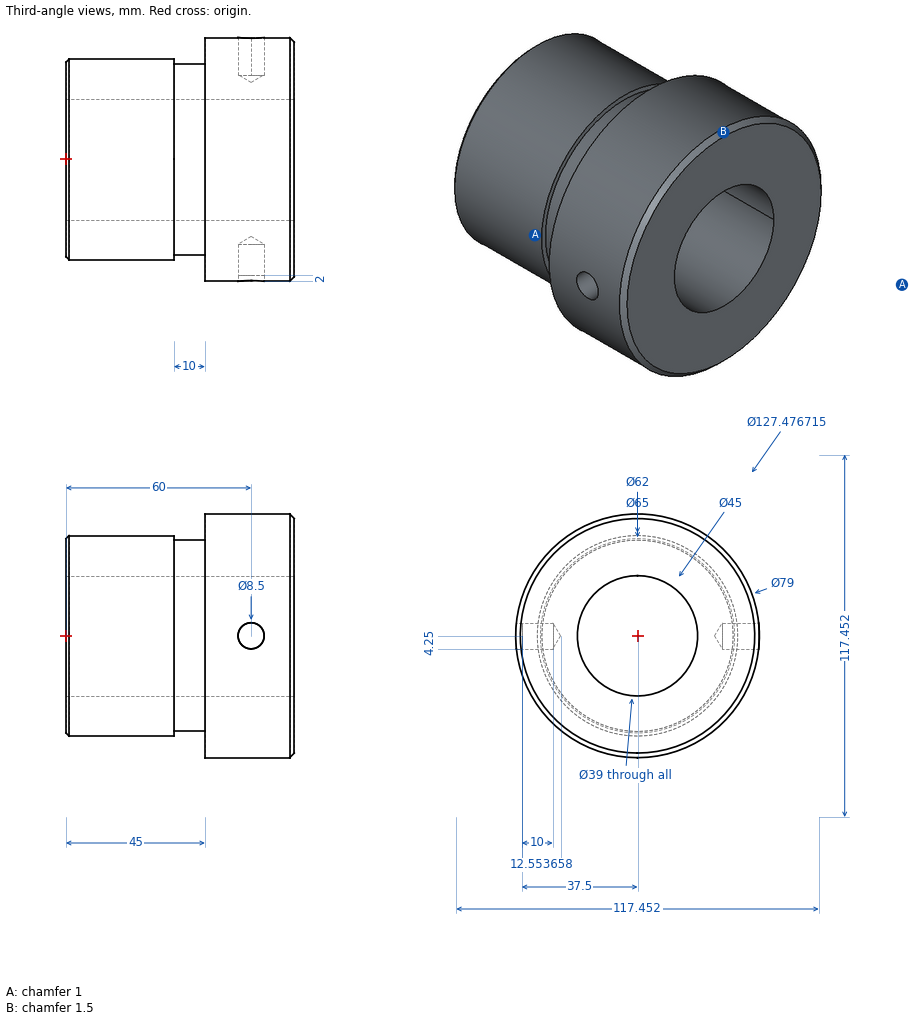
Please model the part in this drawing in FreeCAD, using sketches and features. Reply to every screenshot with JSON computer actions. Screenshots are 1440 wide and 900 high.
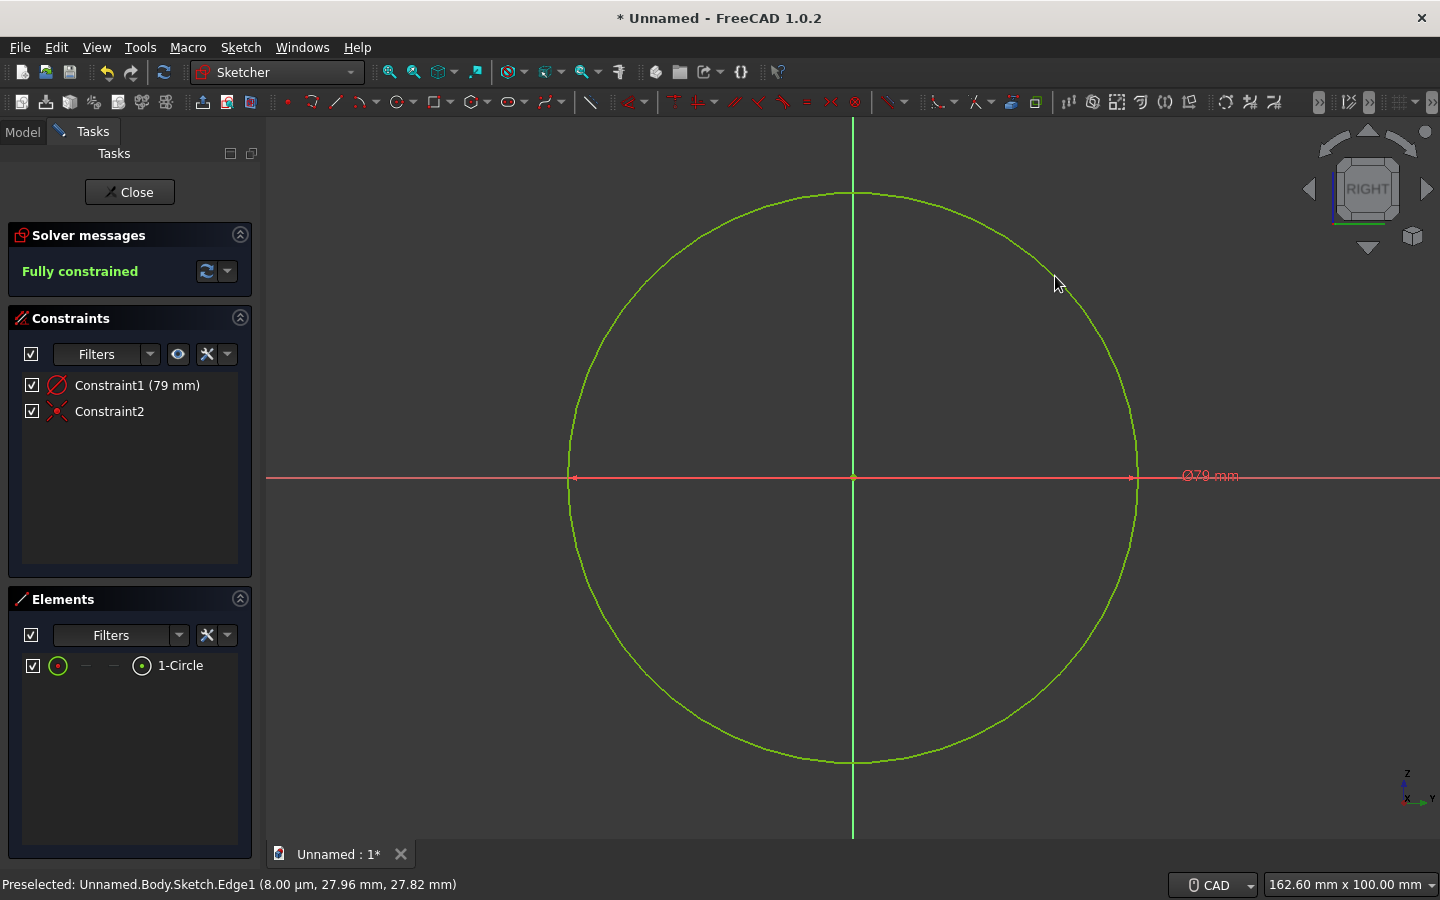
{"action": "left_click", "coordinate": [130, 192]}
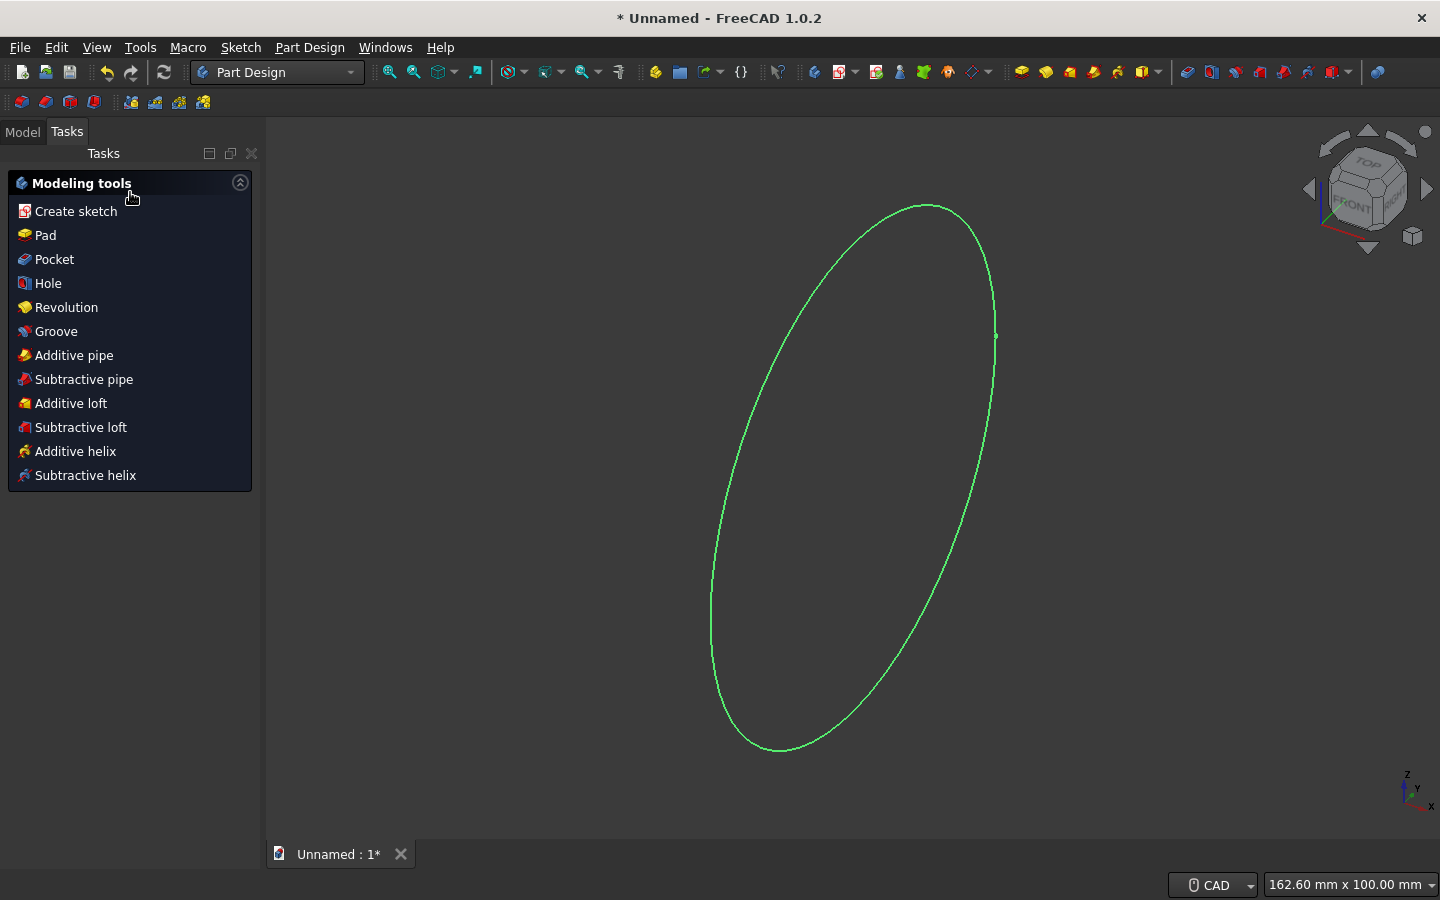
{"action": "left_click", "coordinate": [1022, 72]}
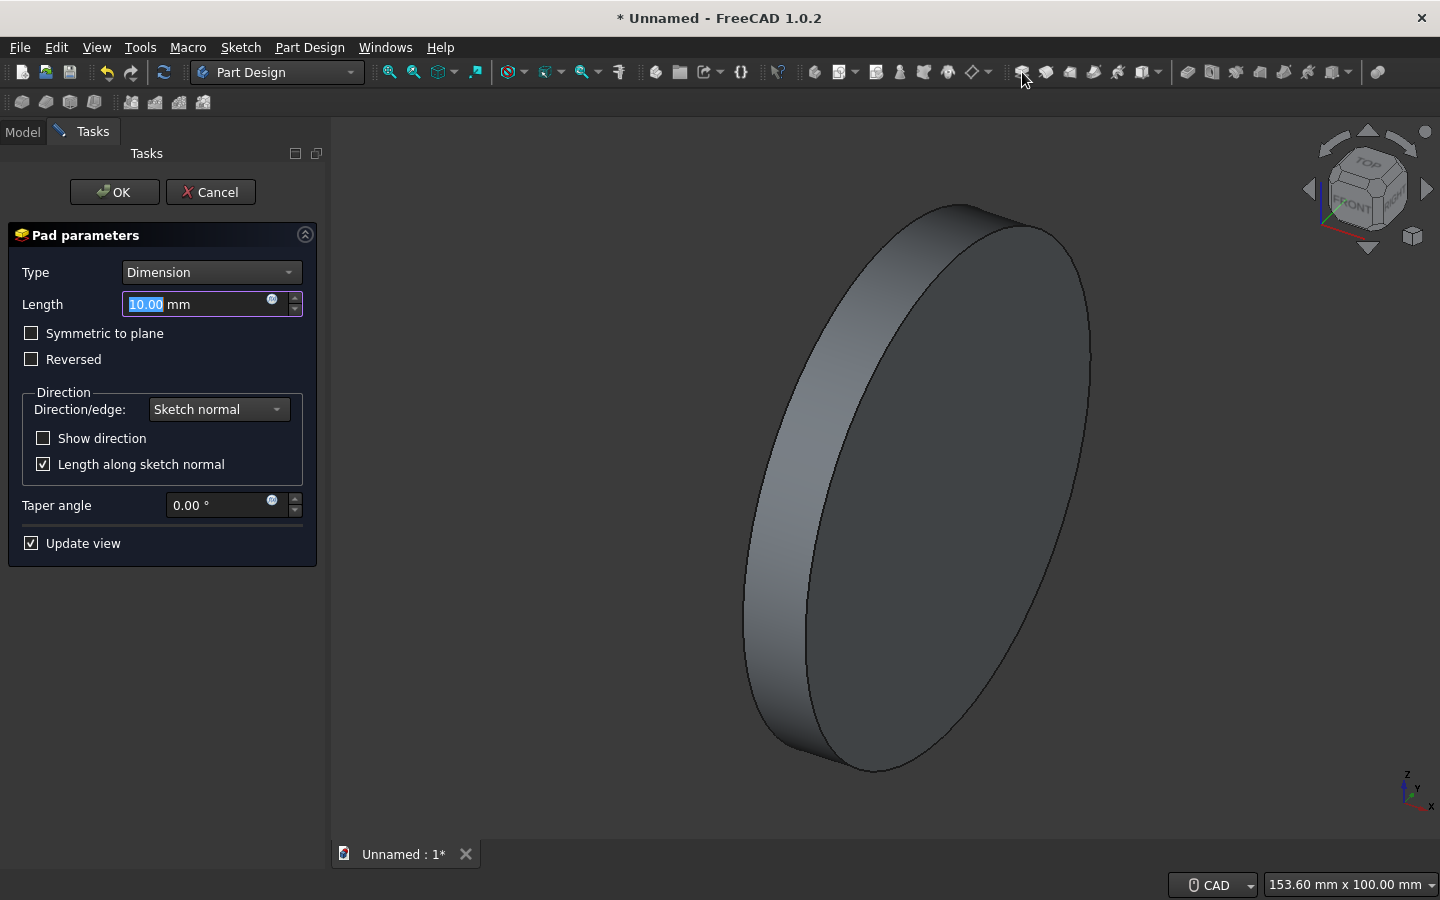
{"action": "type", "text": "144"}
{"action": "key", "text": "Tab"}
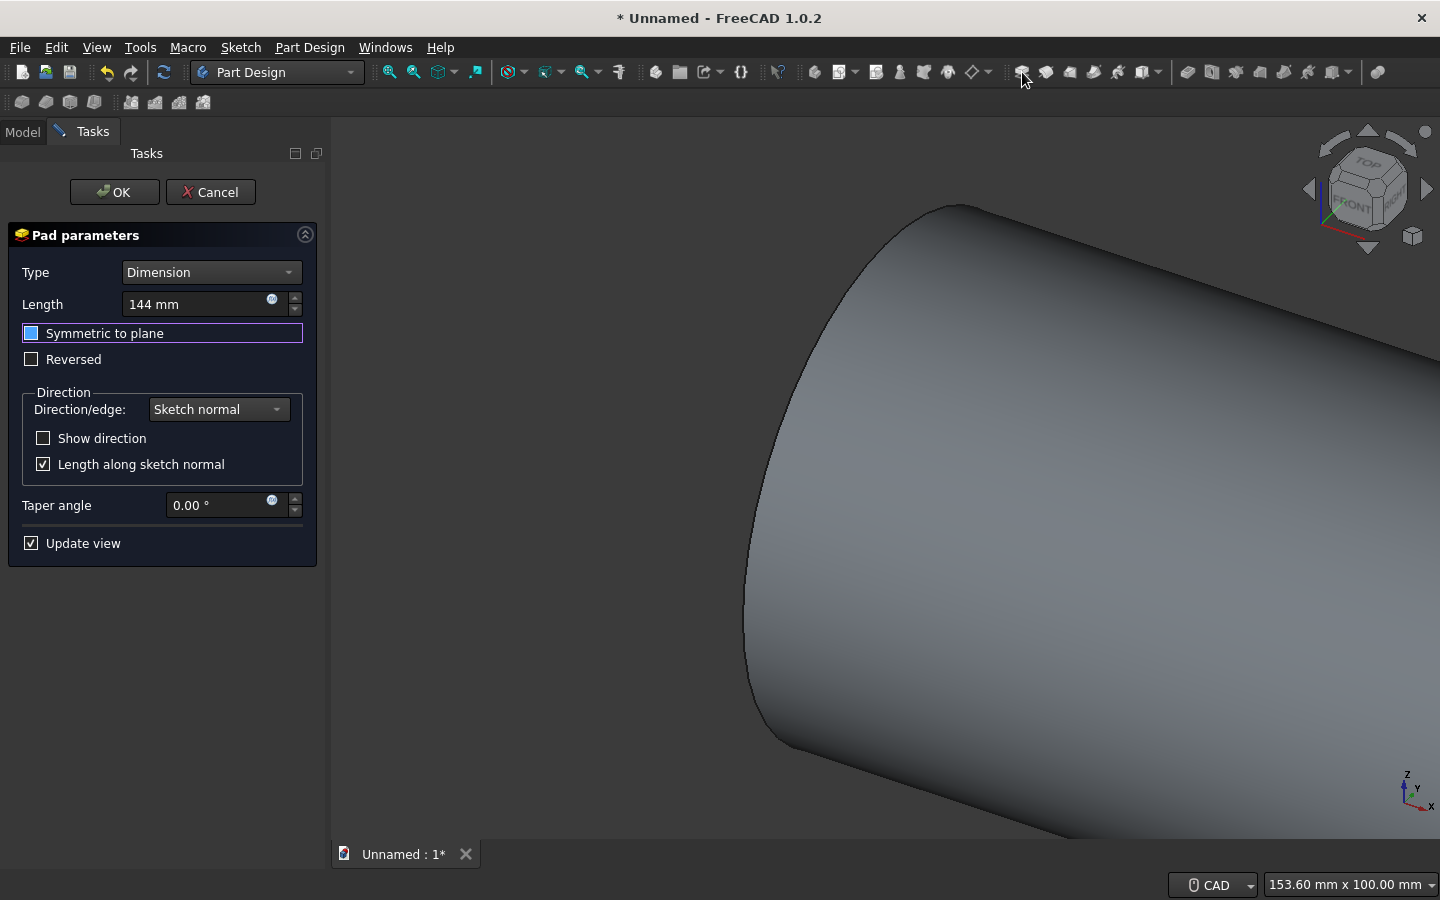
{"action": "left_click", "coordinate": [115, 192]}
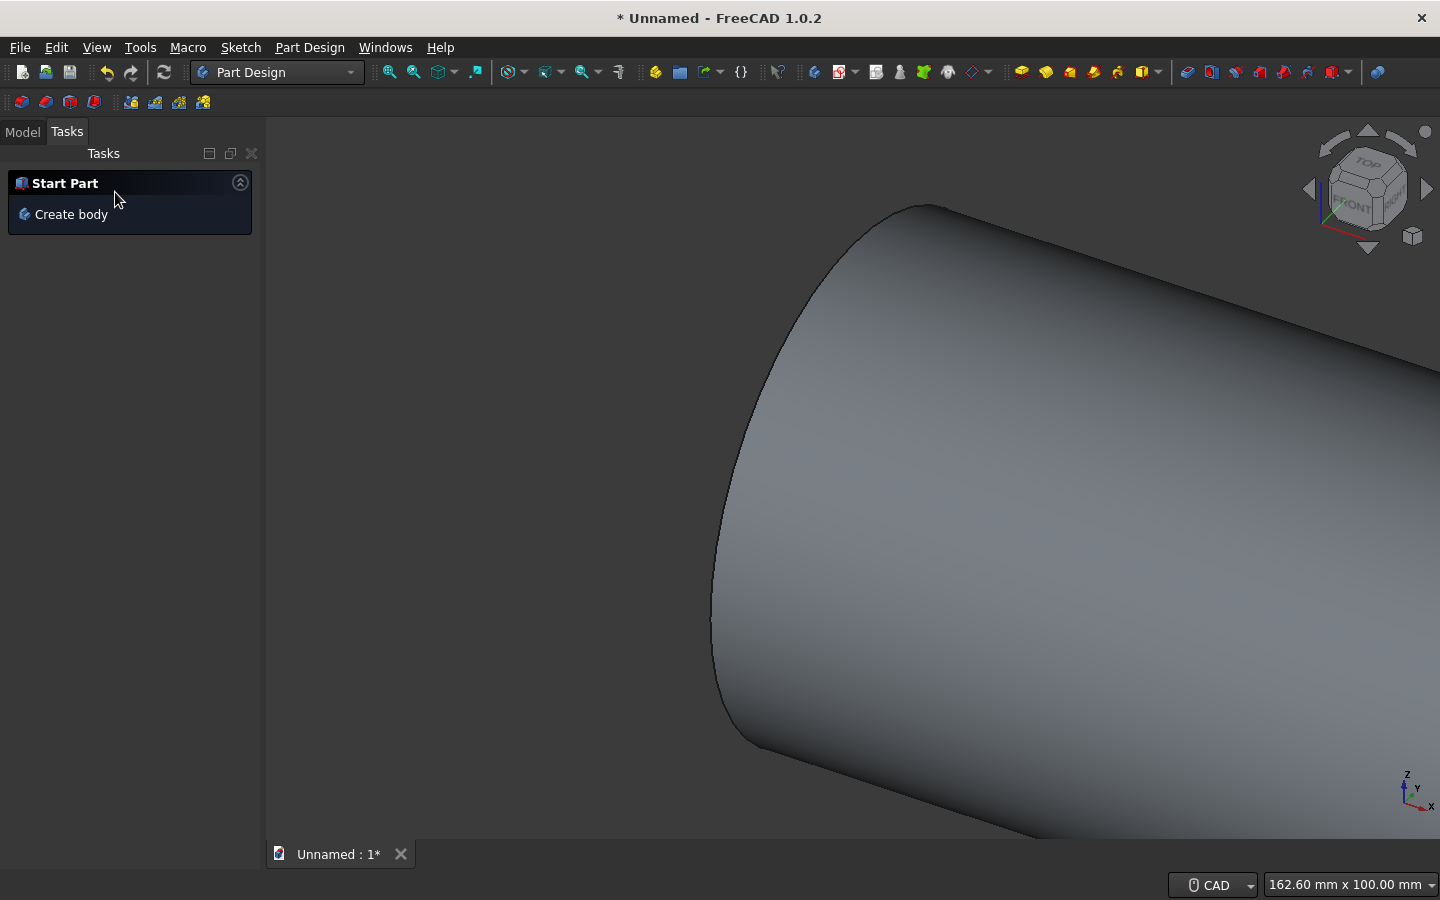
{"action": "key", "text": "v f"}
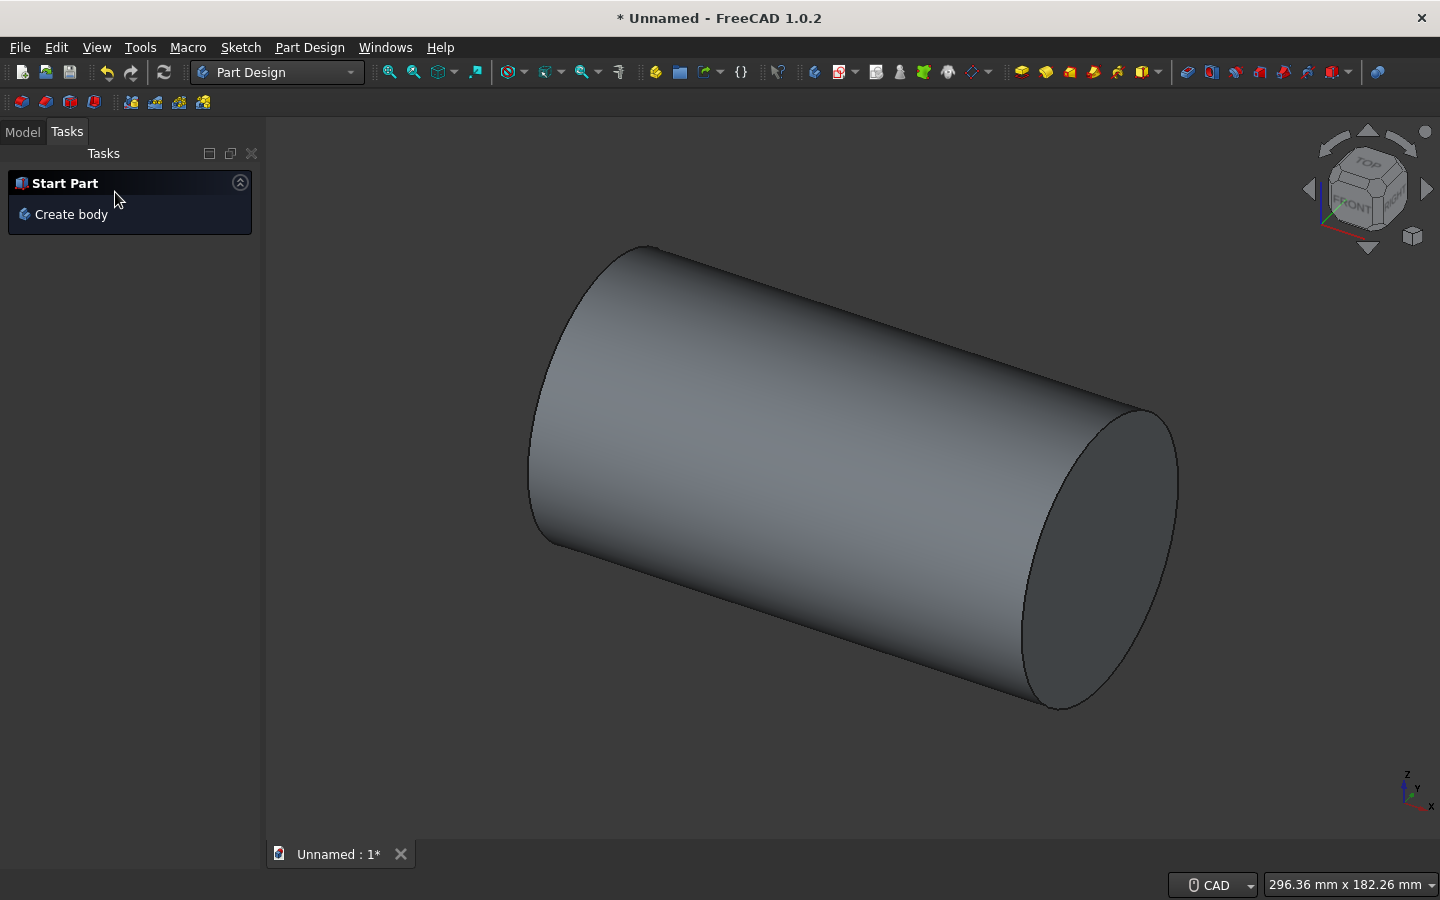
{"action": "left_click", "coordinate": [1100, 559]}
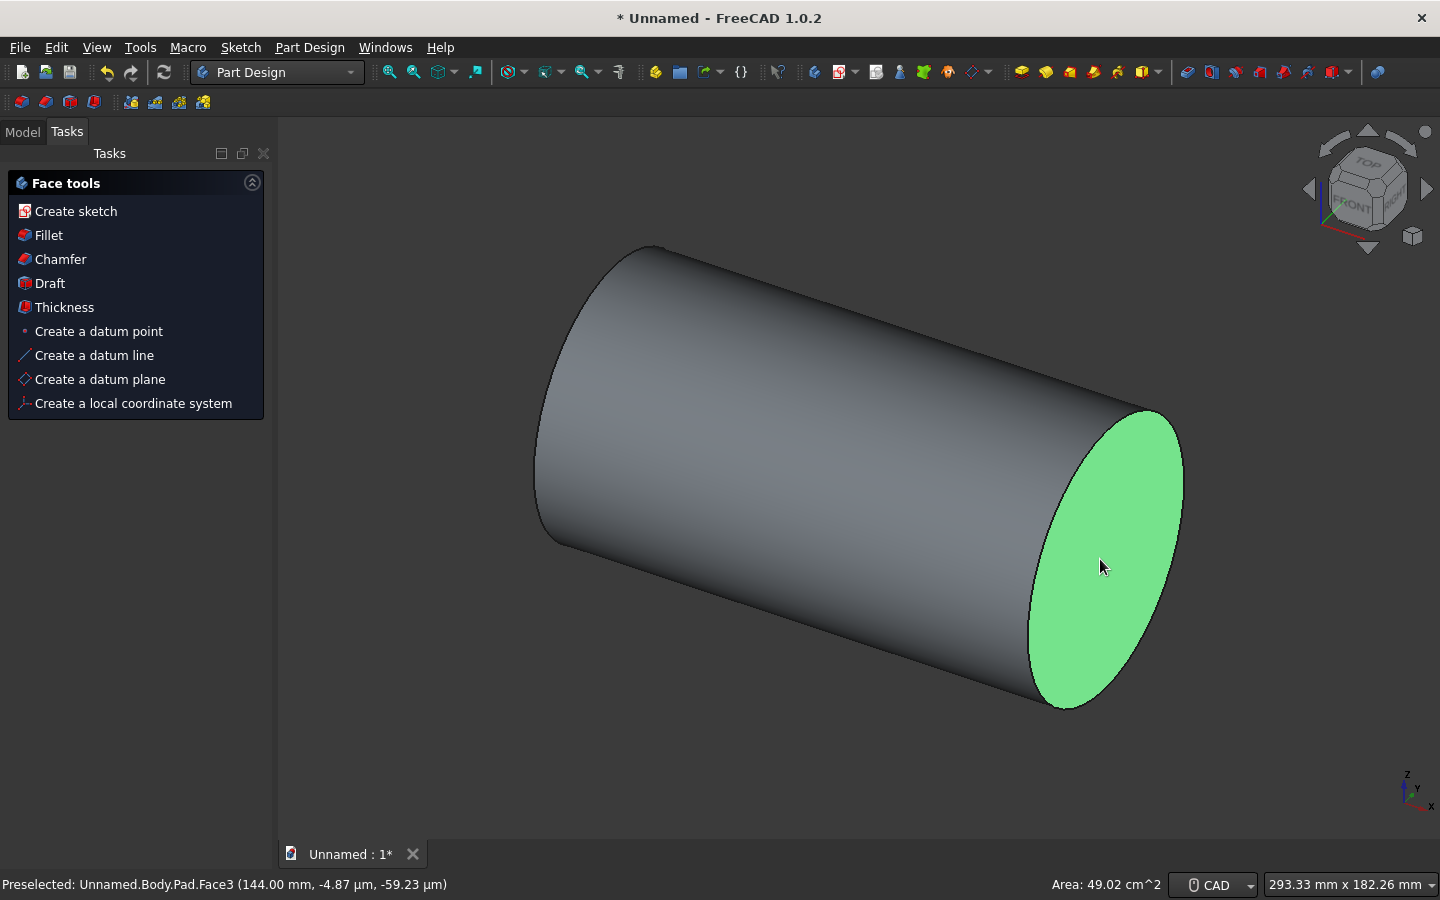
{"action": "left_click", "coordinate": [840, 72]}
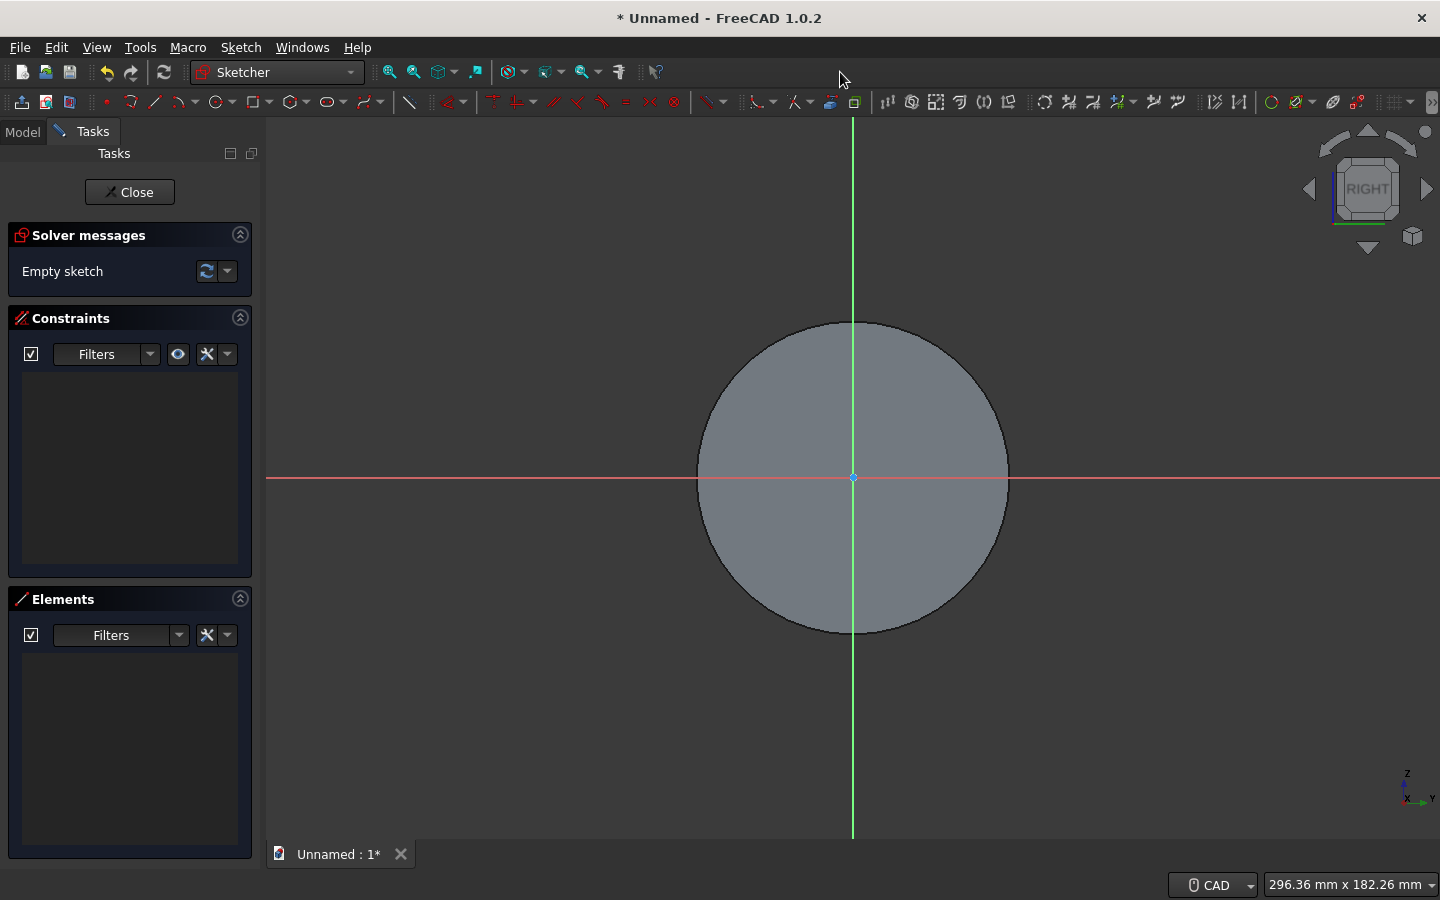
{"action": "key", "text": "g v"}